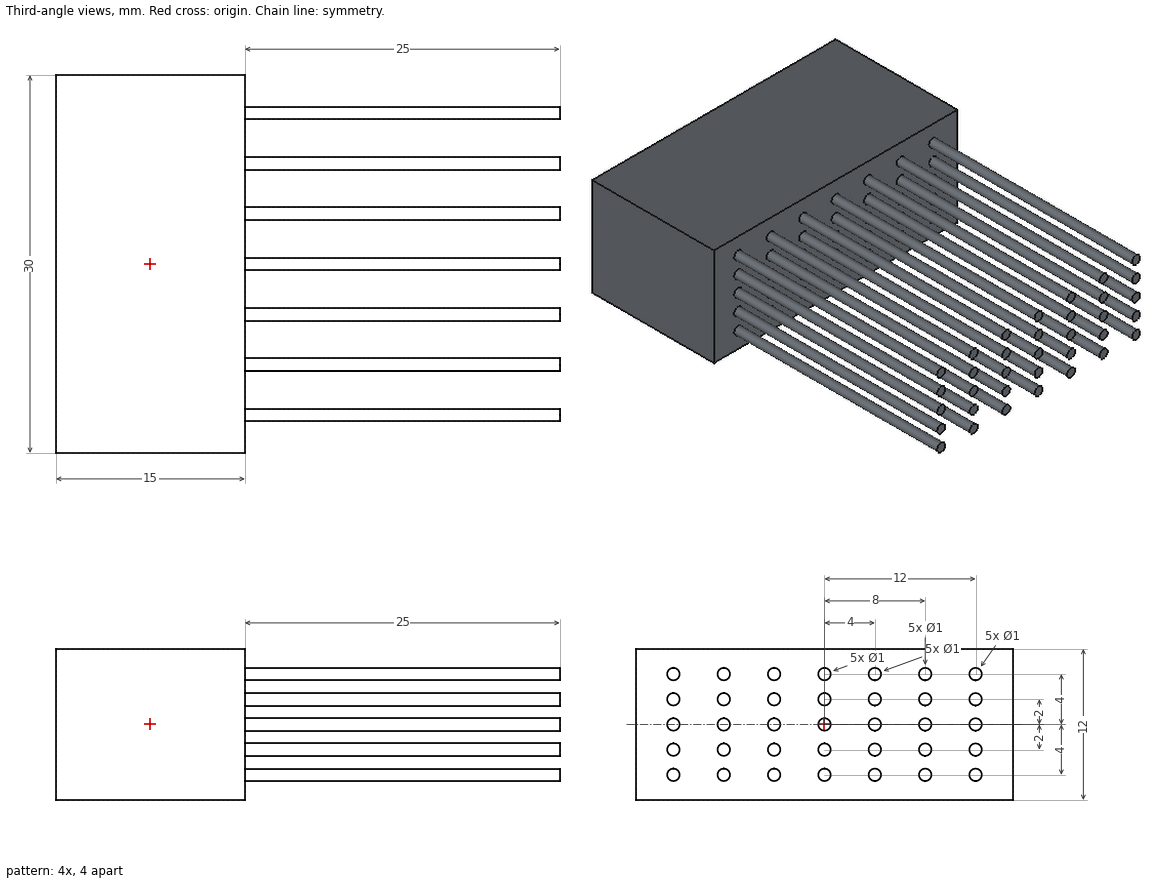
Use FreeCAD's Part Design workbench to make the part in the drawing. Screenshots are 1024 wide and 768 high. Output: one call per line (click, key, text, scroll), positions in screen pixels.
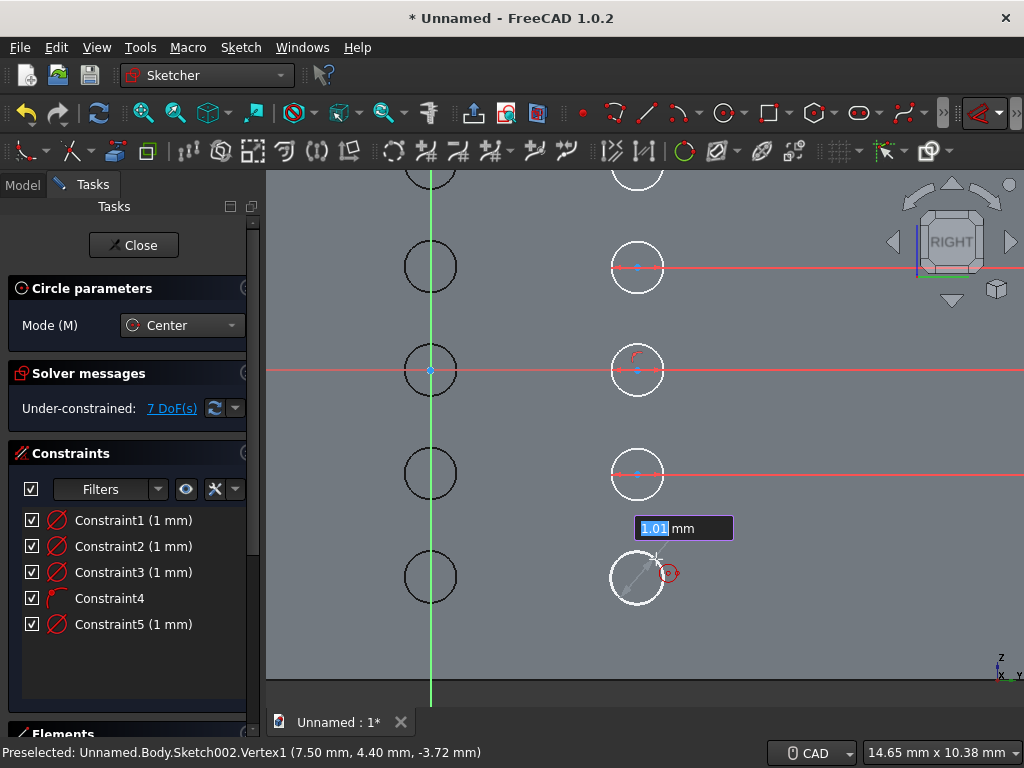
text(1)
key(Return)
key(Escape)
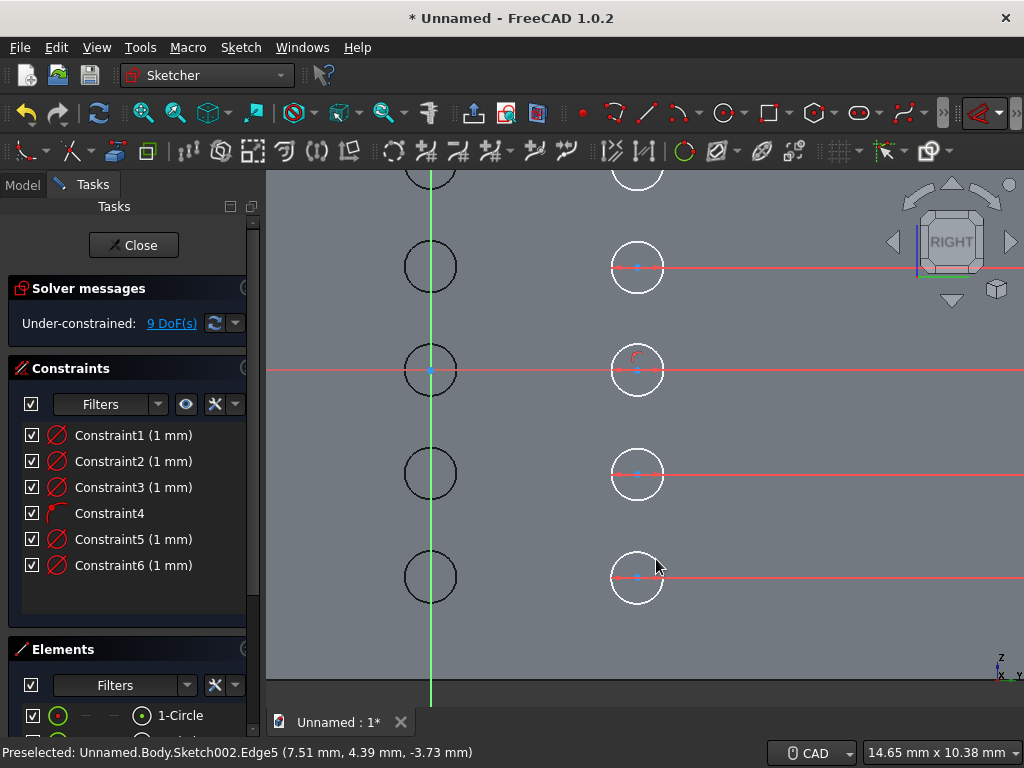
click(637, 268)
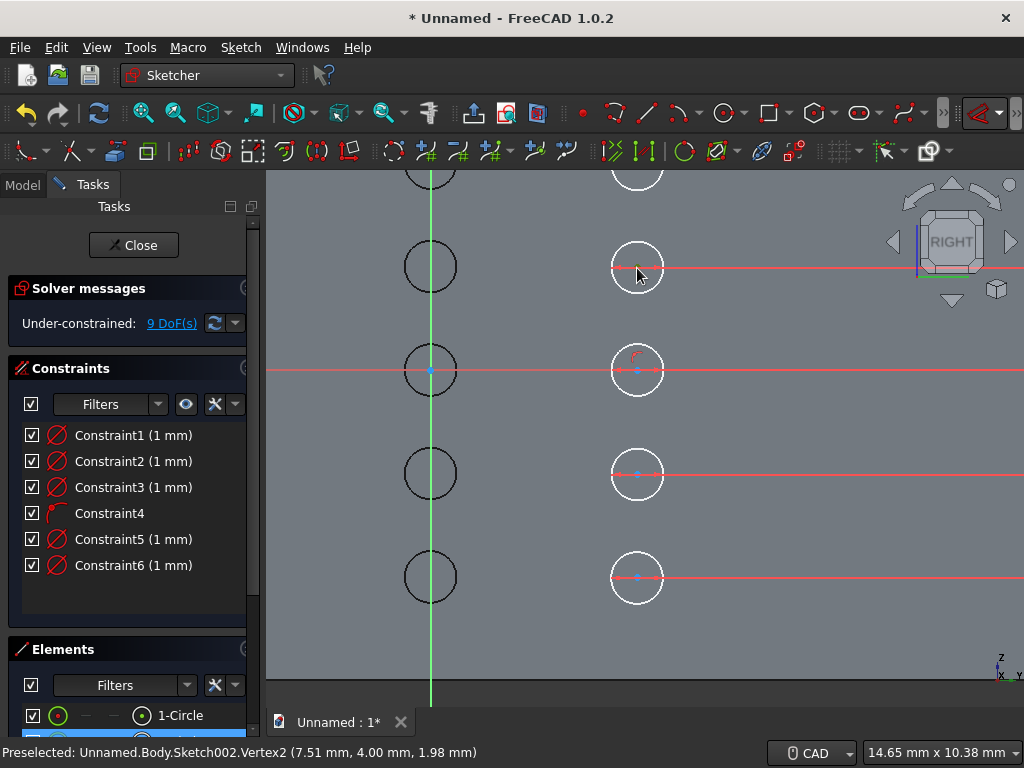
click(637, 475)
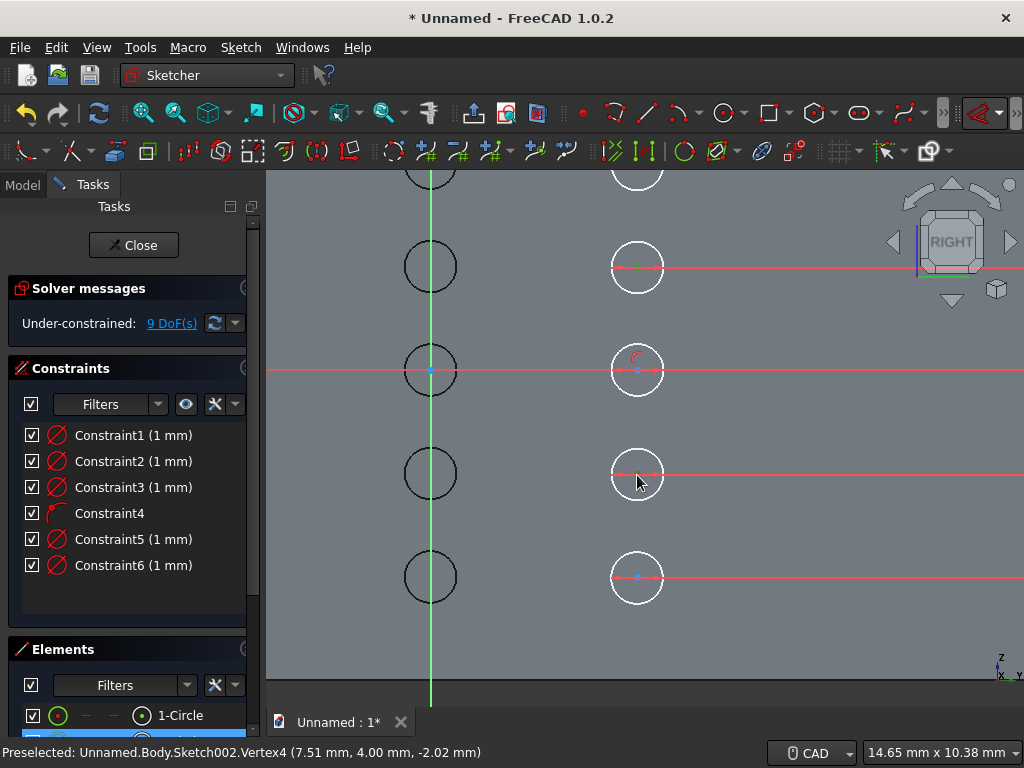
click(334, 370)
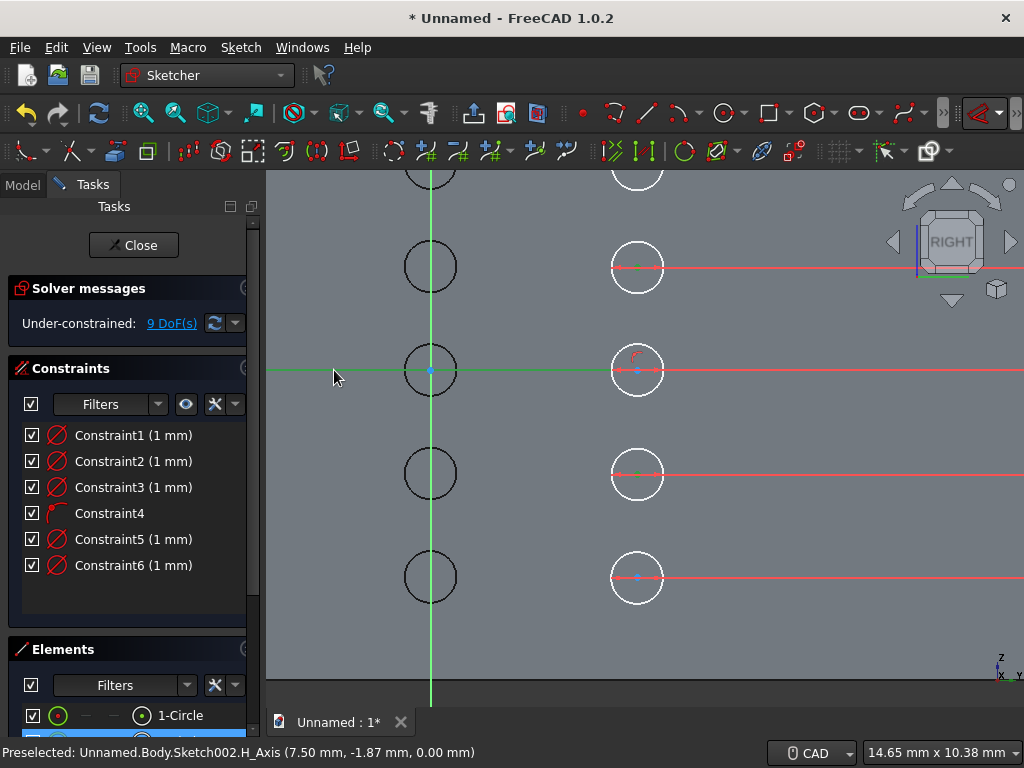
key(s)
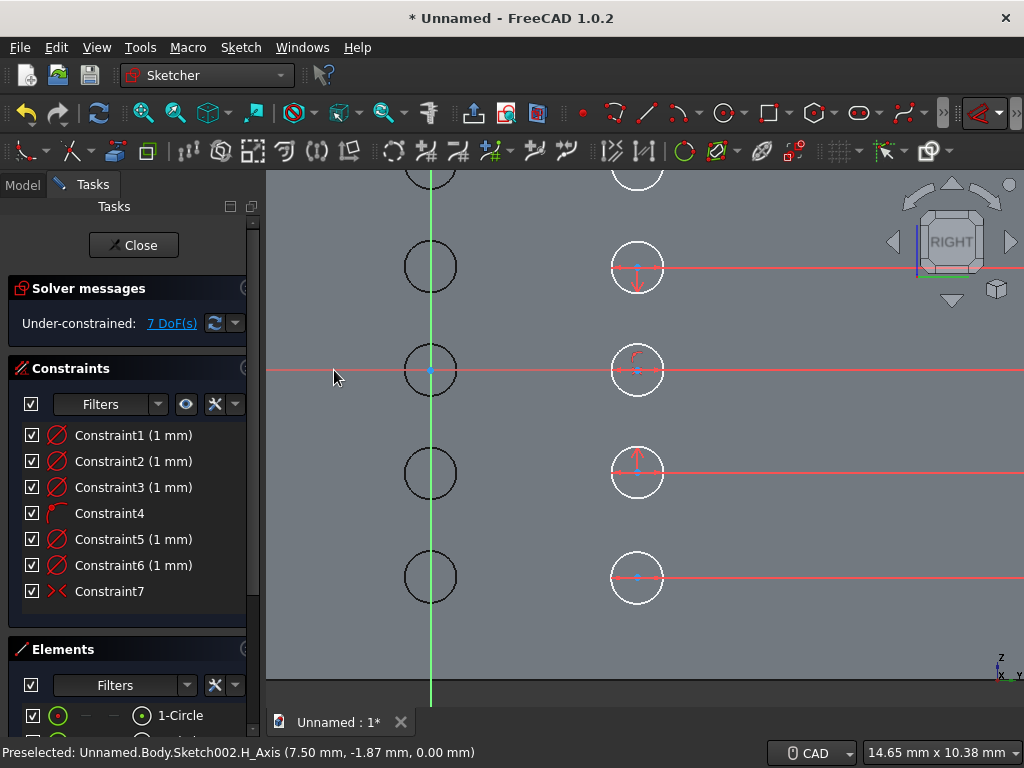
scroll(637, 578, down, 2)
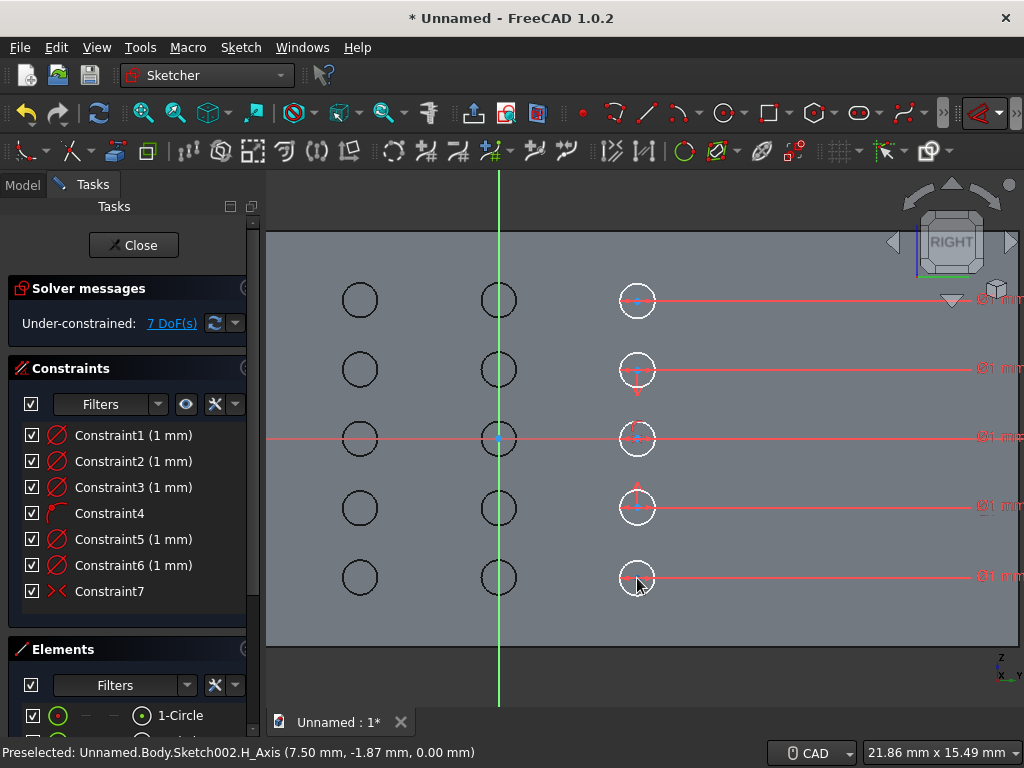
click(637, 301)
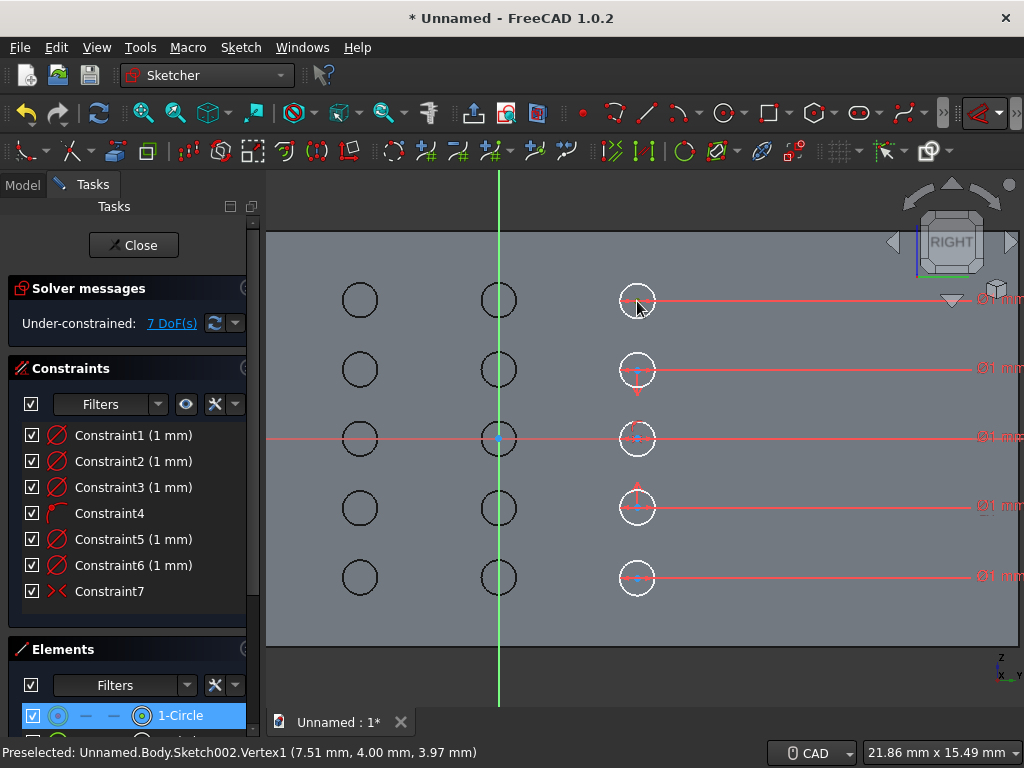
click(637, 578)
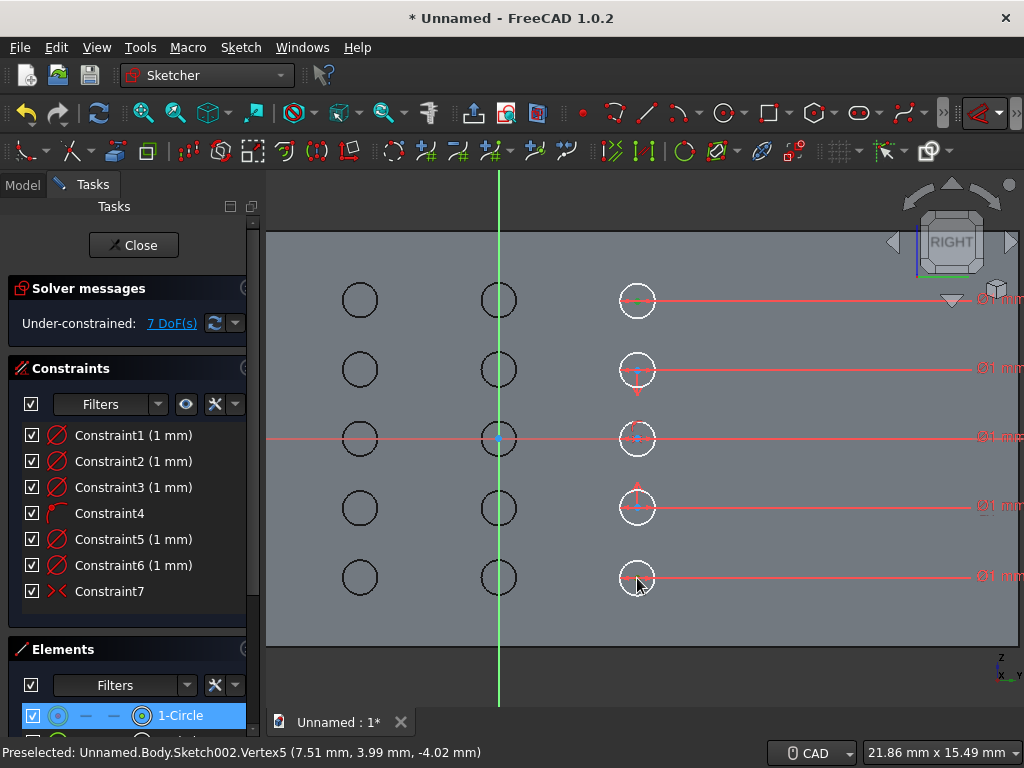
click(334, 439)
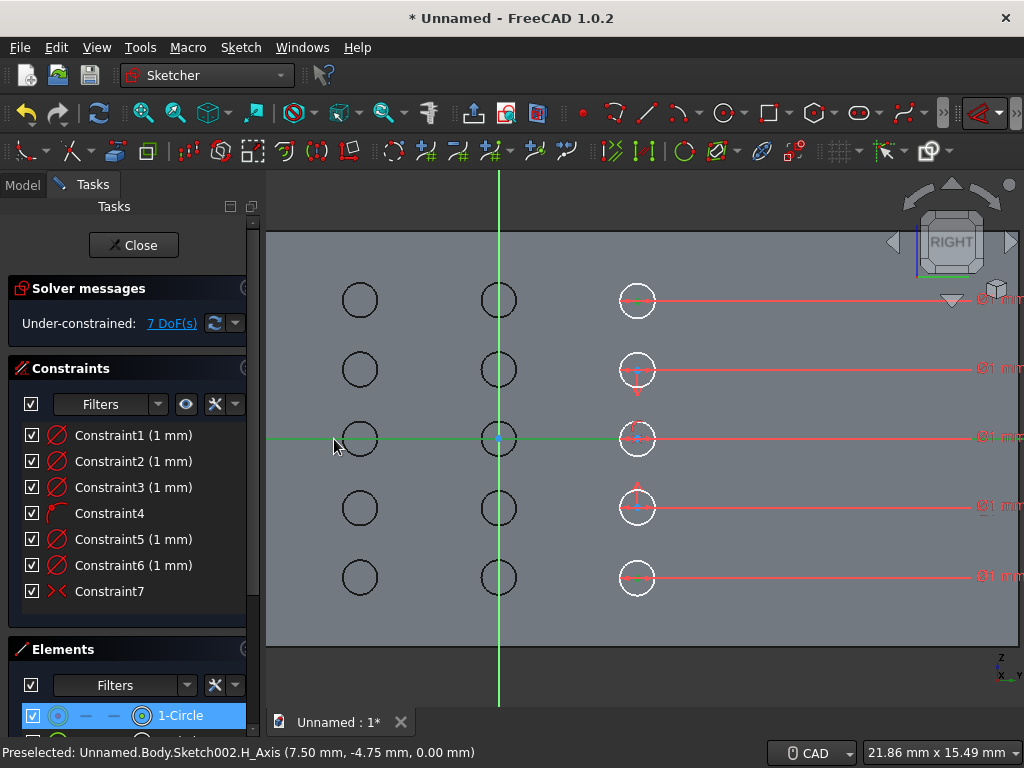
key(s)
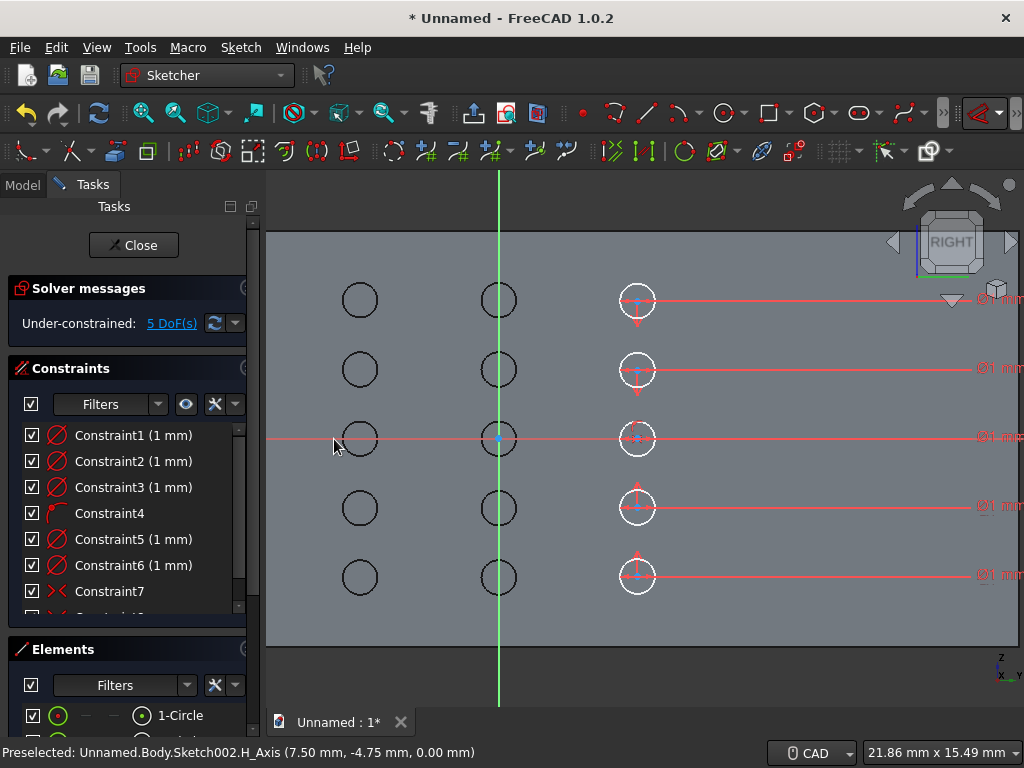
click(637, 301)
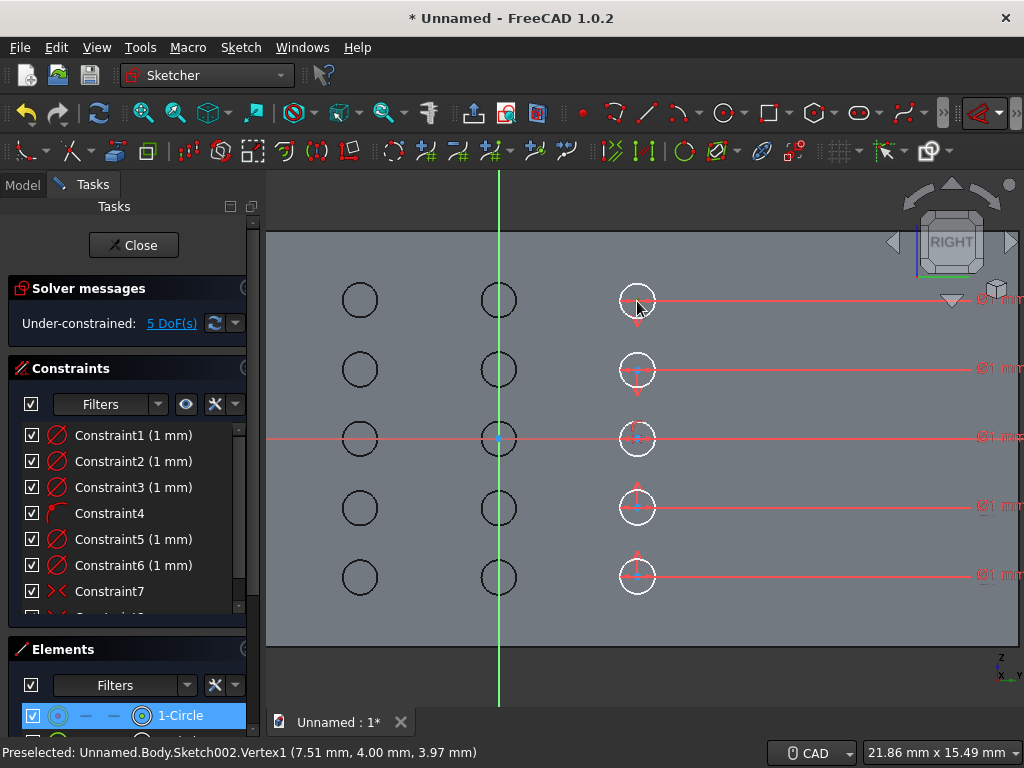
key(l)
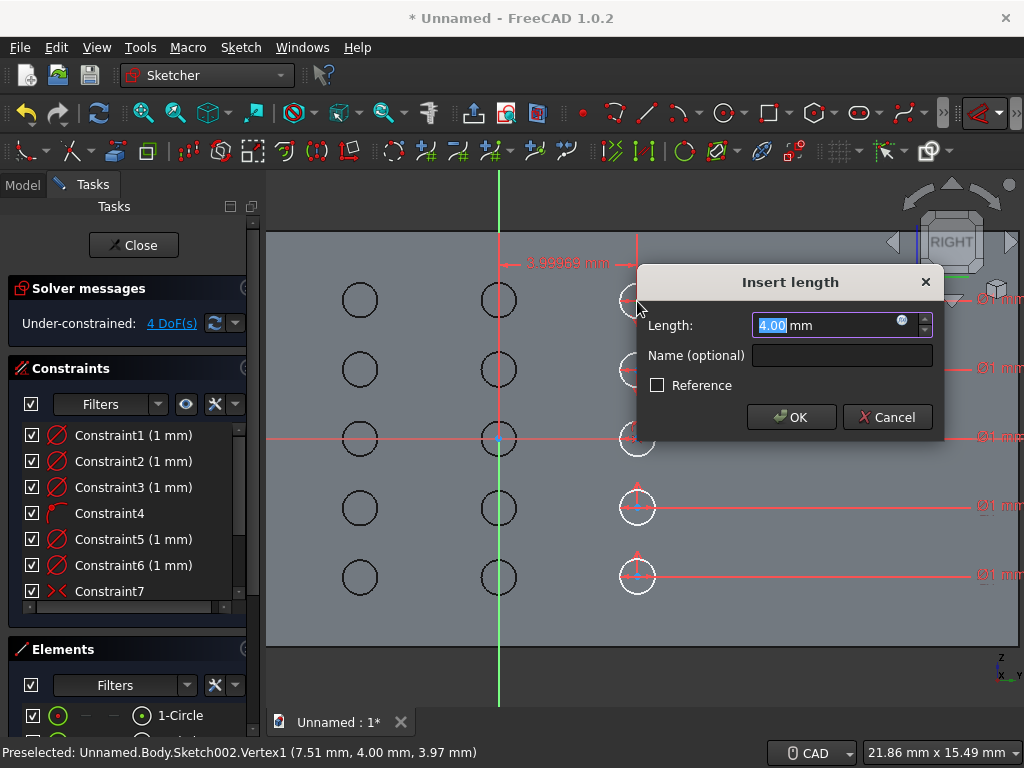
text(4)
key(Return)